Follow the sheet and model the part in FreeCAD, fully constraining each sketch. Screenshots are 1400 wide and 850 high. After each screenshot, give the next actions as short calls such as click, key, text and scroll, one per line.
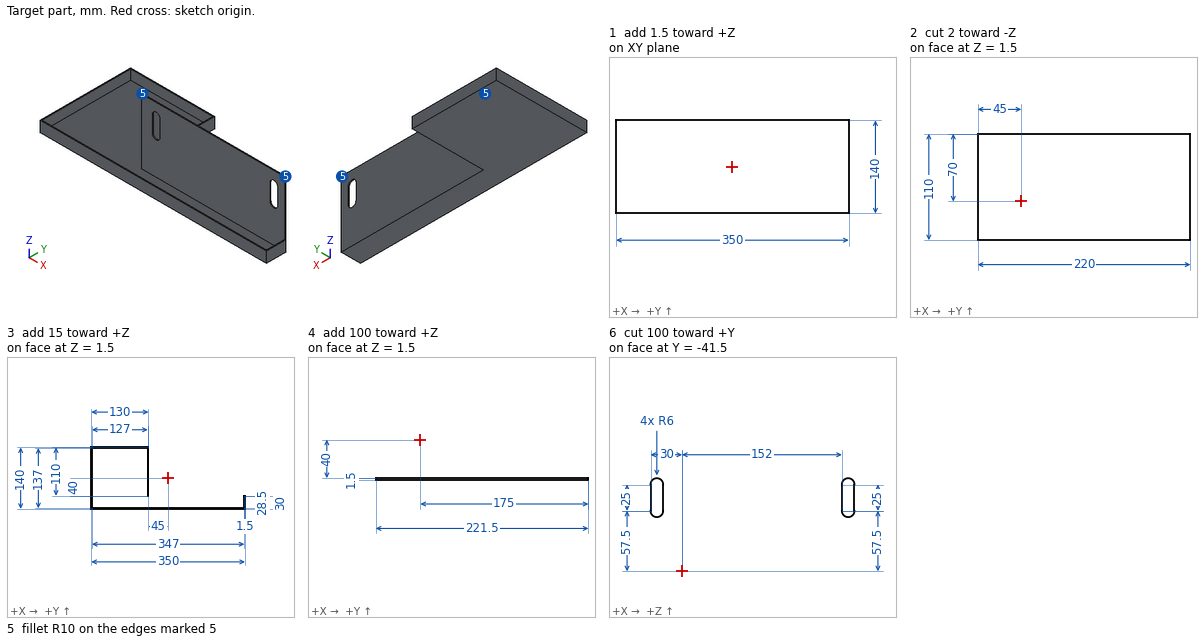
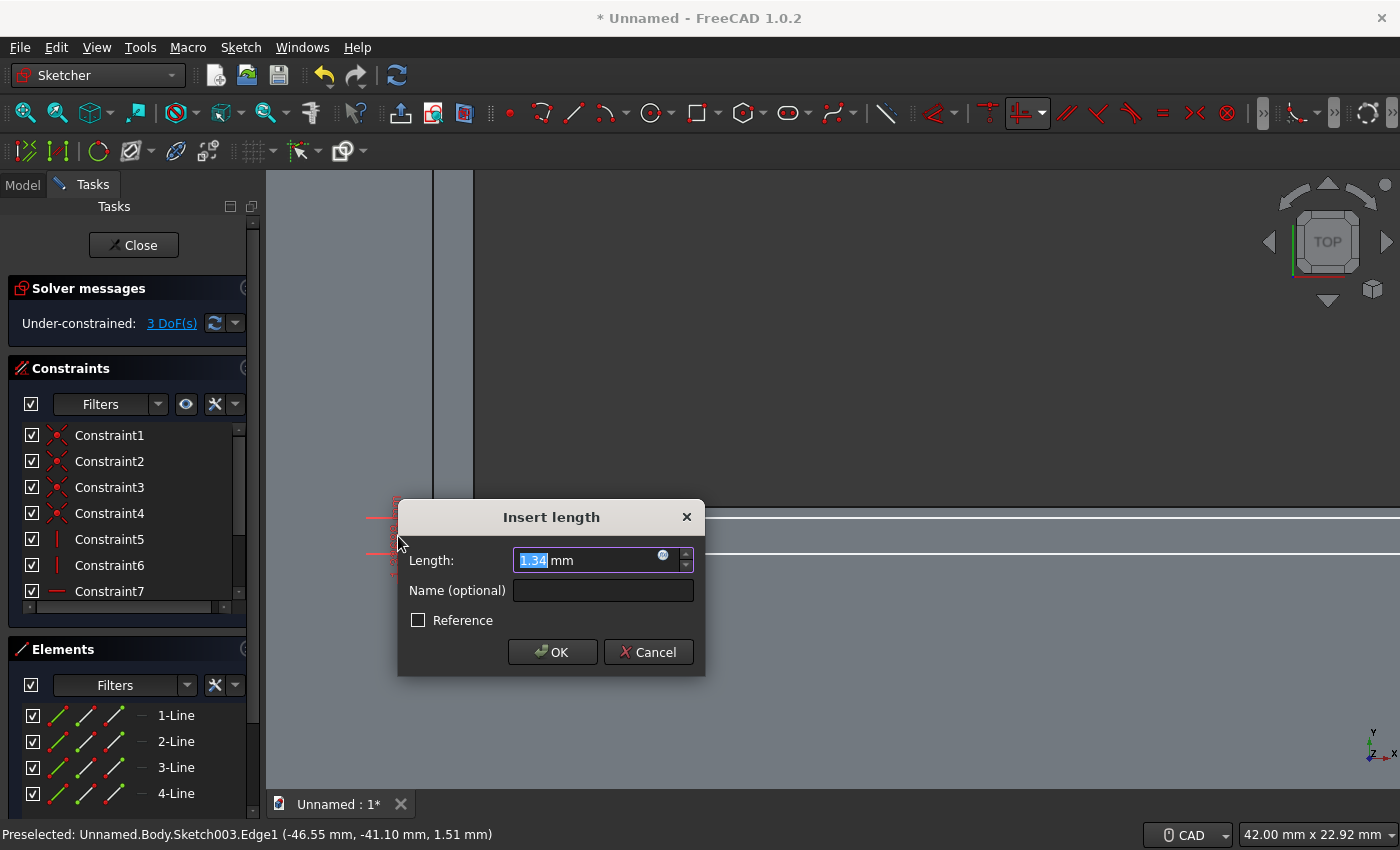
text(1.5)
key(Return)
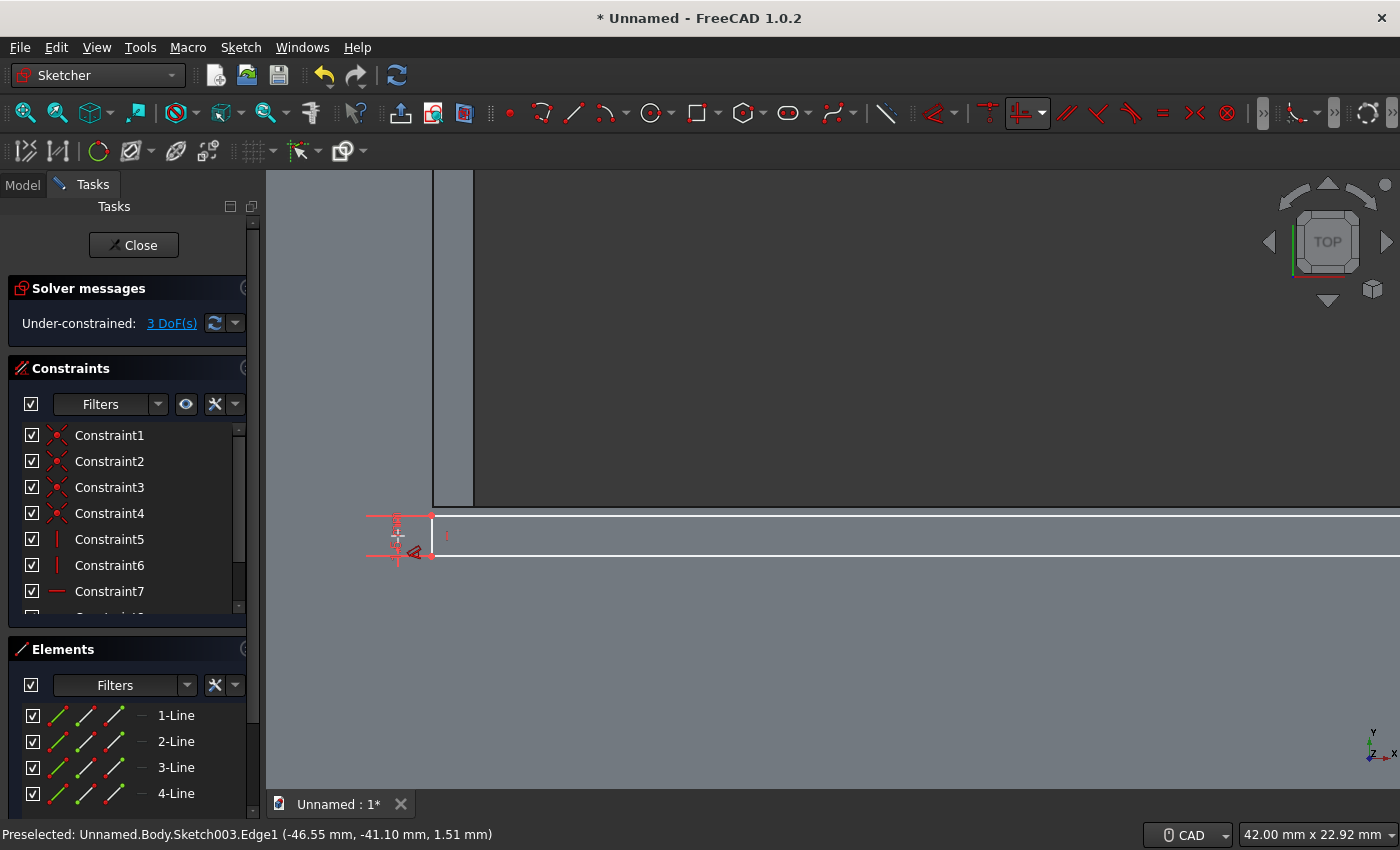
scroll(433, 541, down, 11)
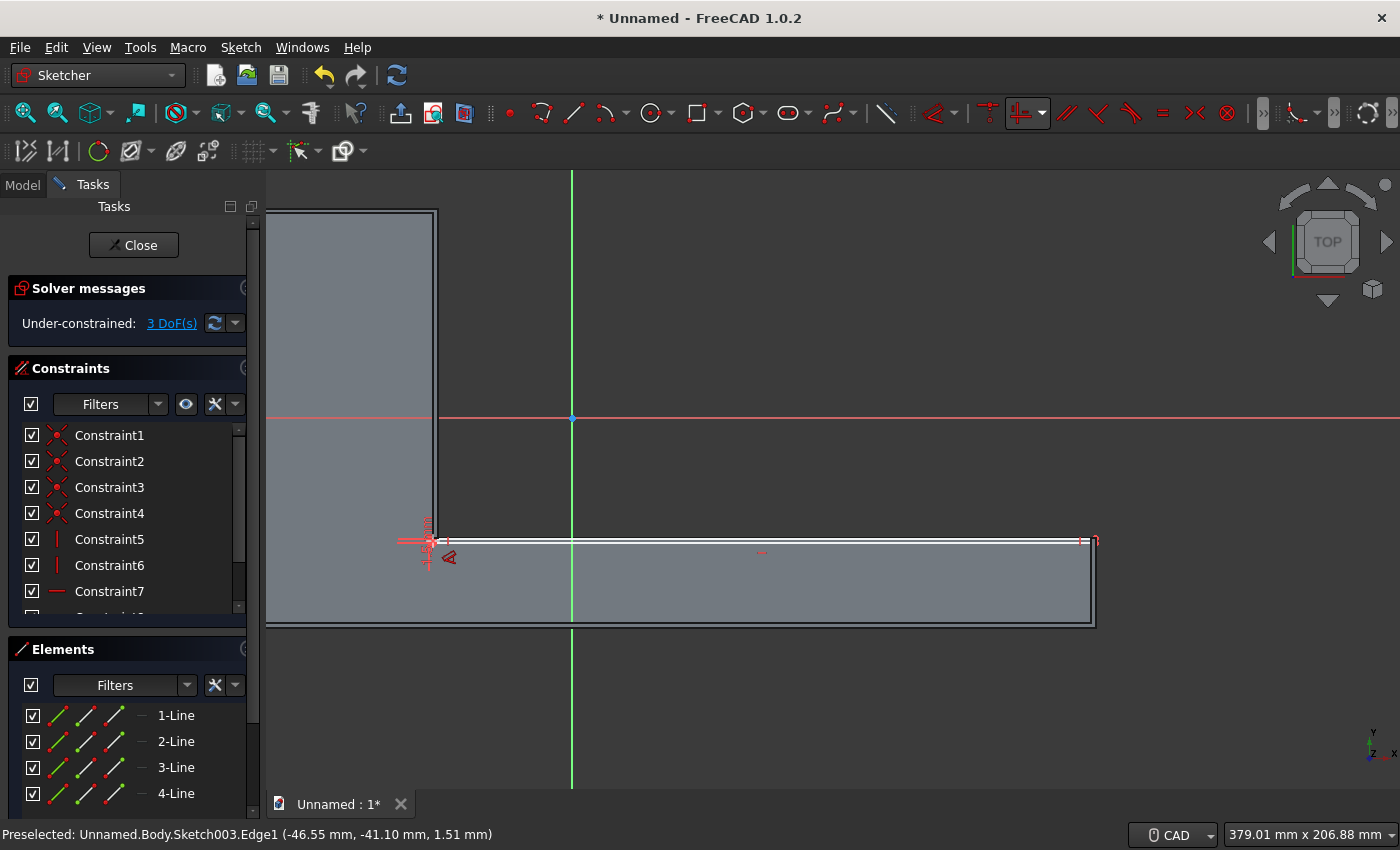
scroll(433, 539, up, 6)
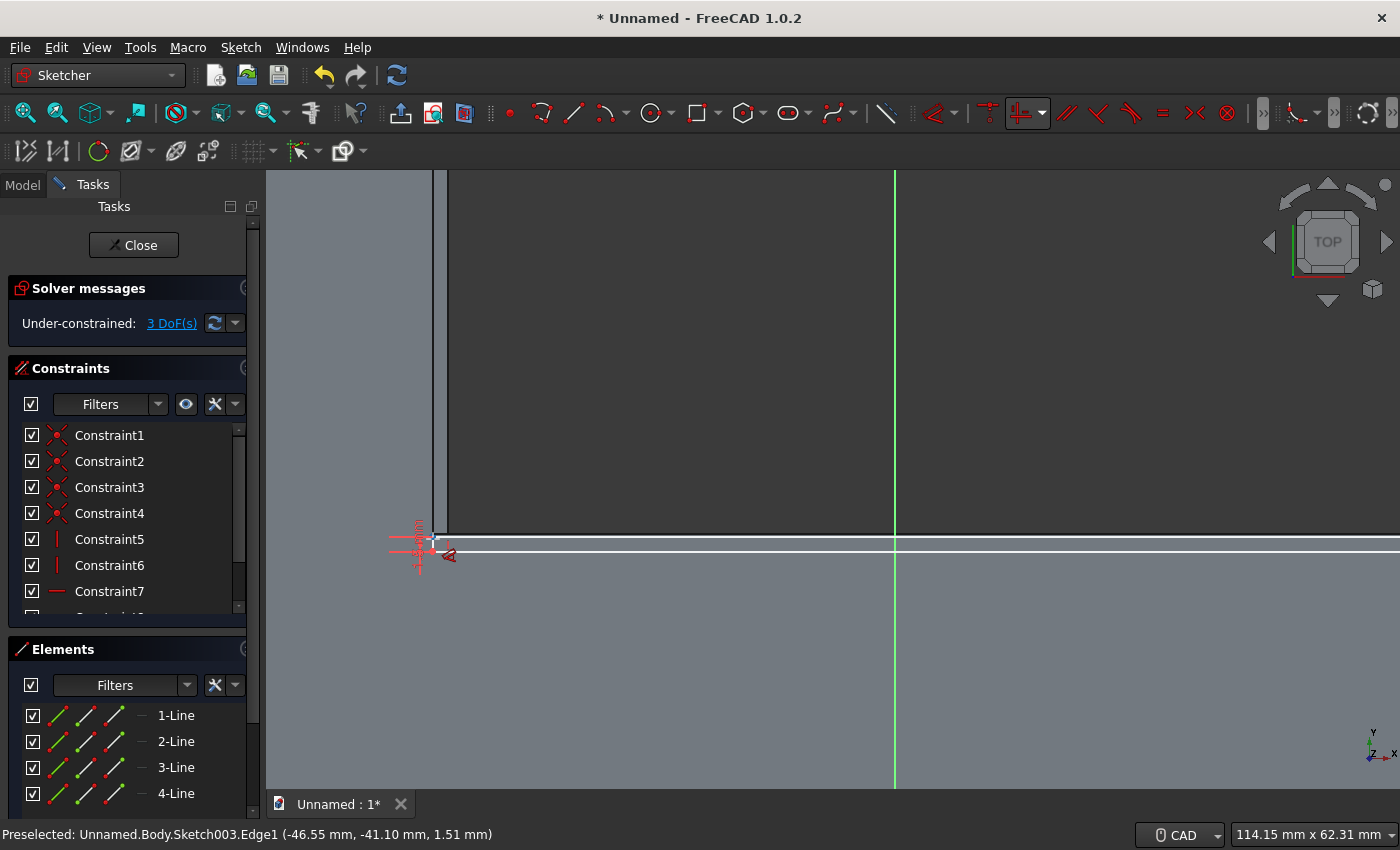
click(433, 537)
click(399, 367)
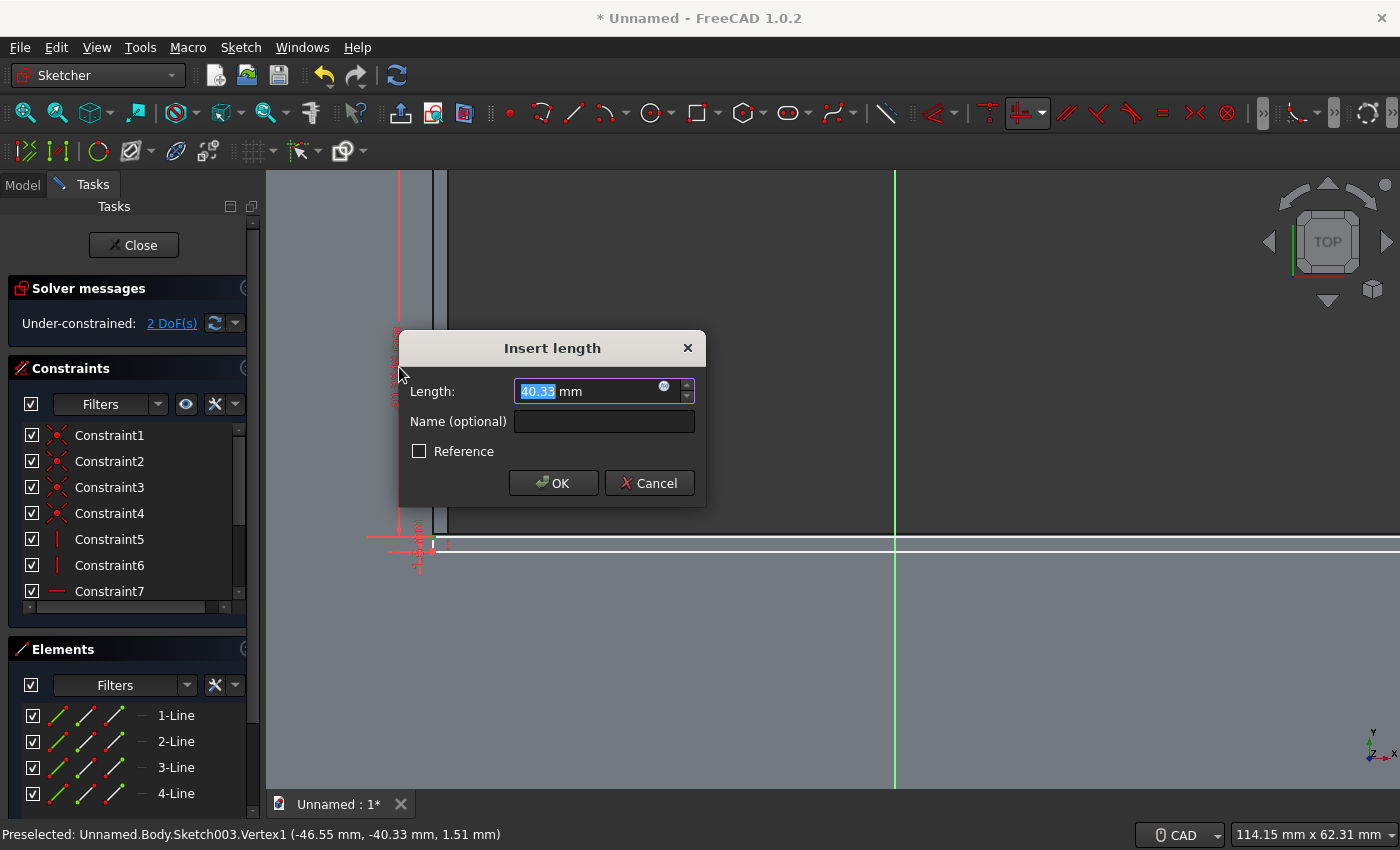
text(40)
key(Return)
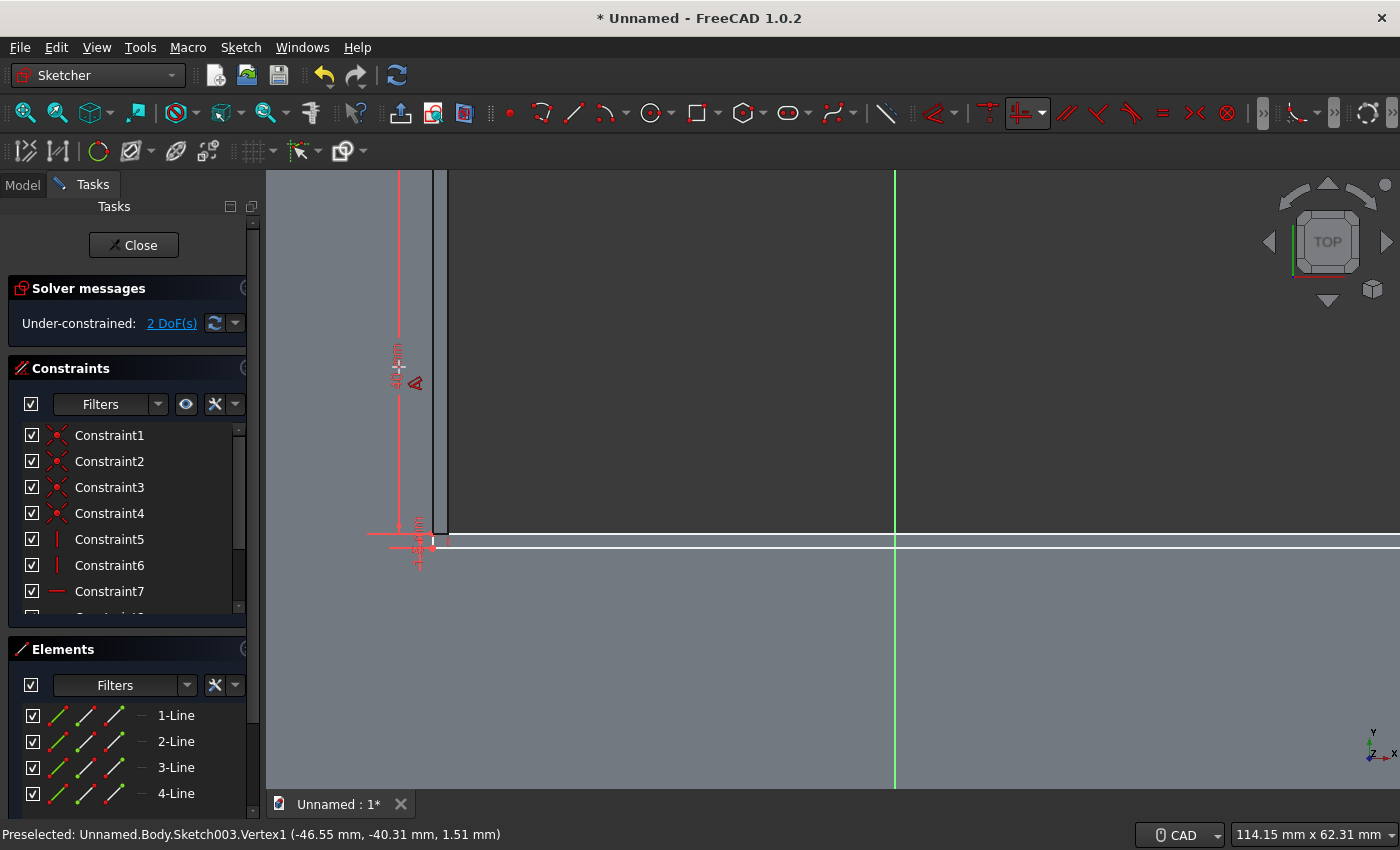
scroll(433, 539, down, 6)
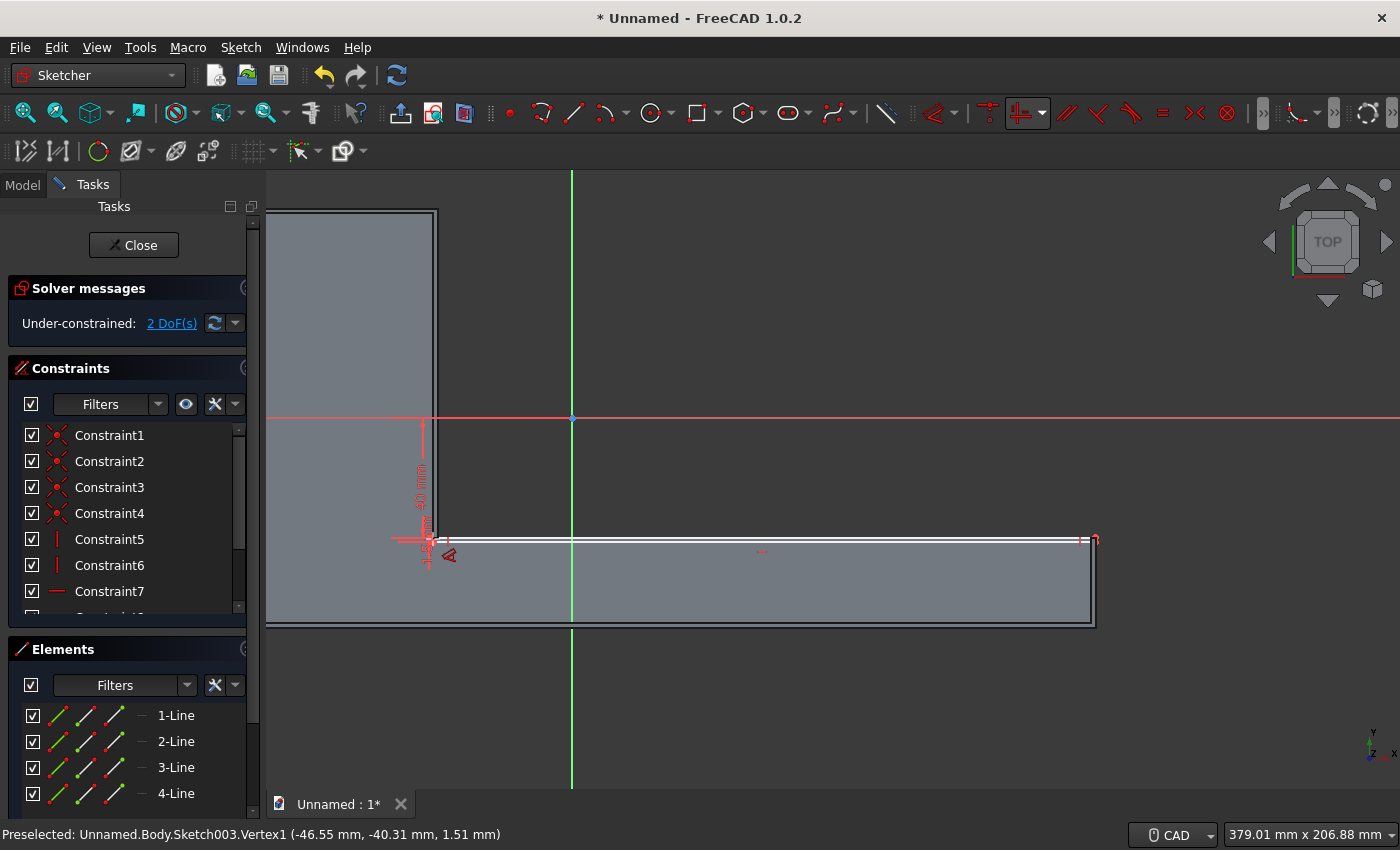
scroll(1096, 542, up, 6)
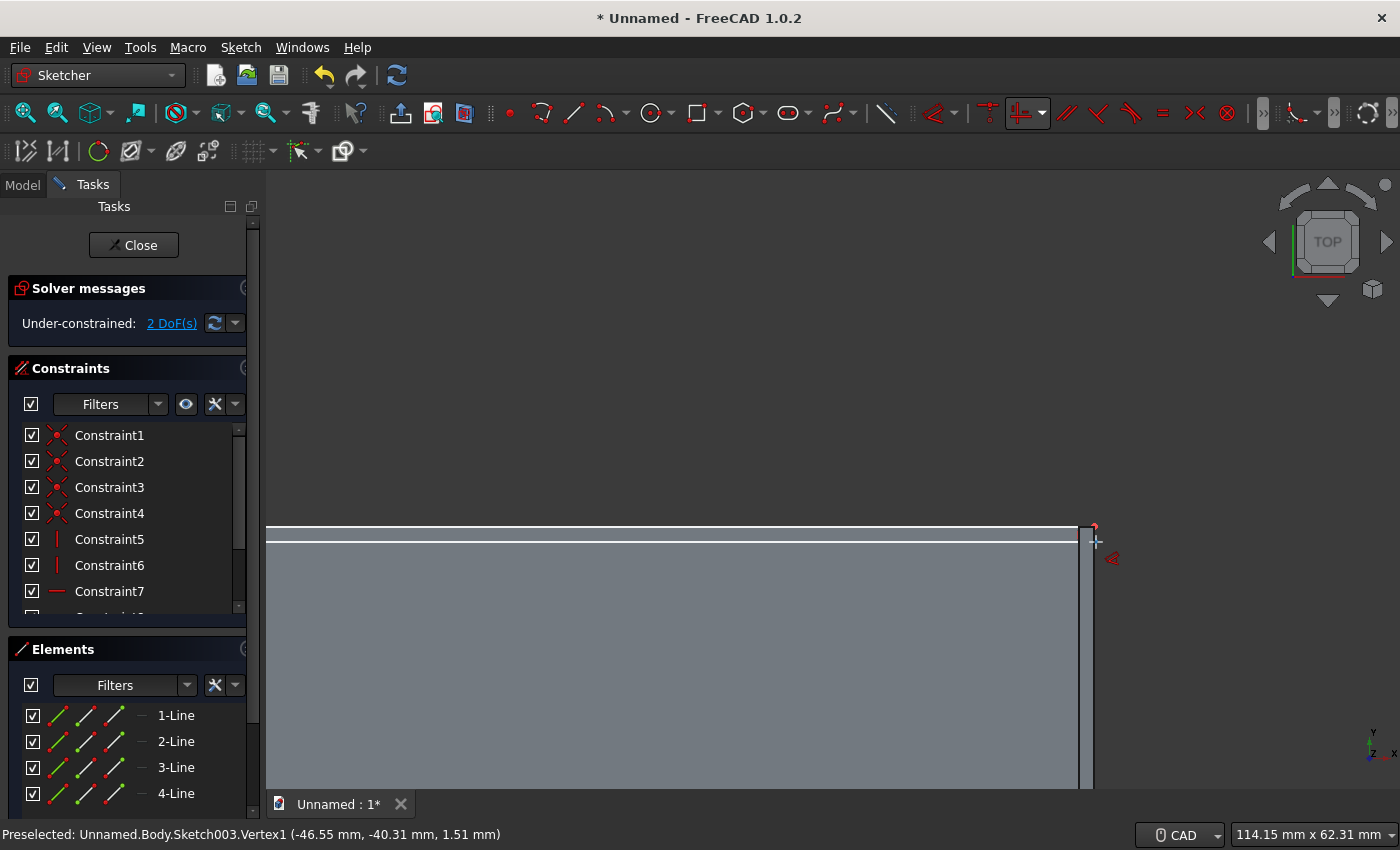
click(1094, 542)
click(694, 576)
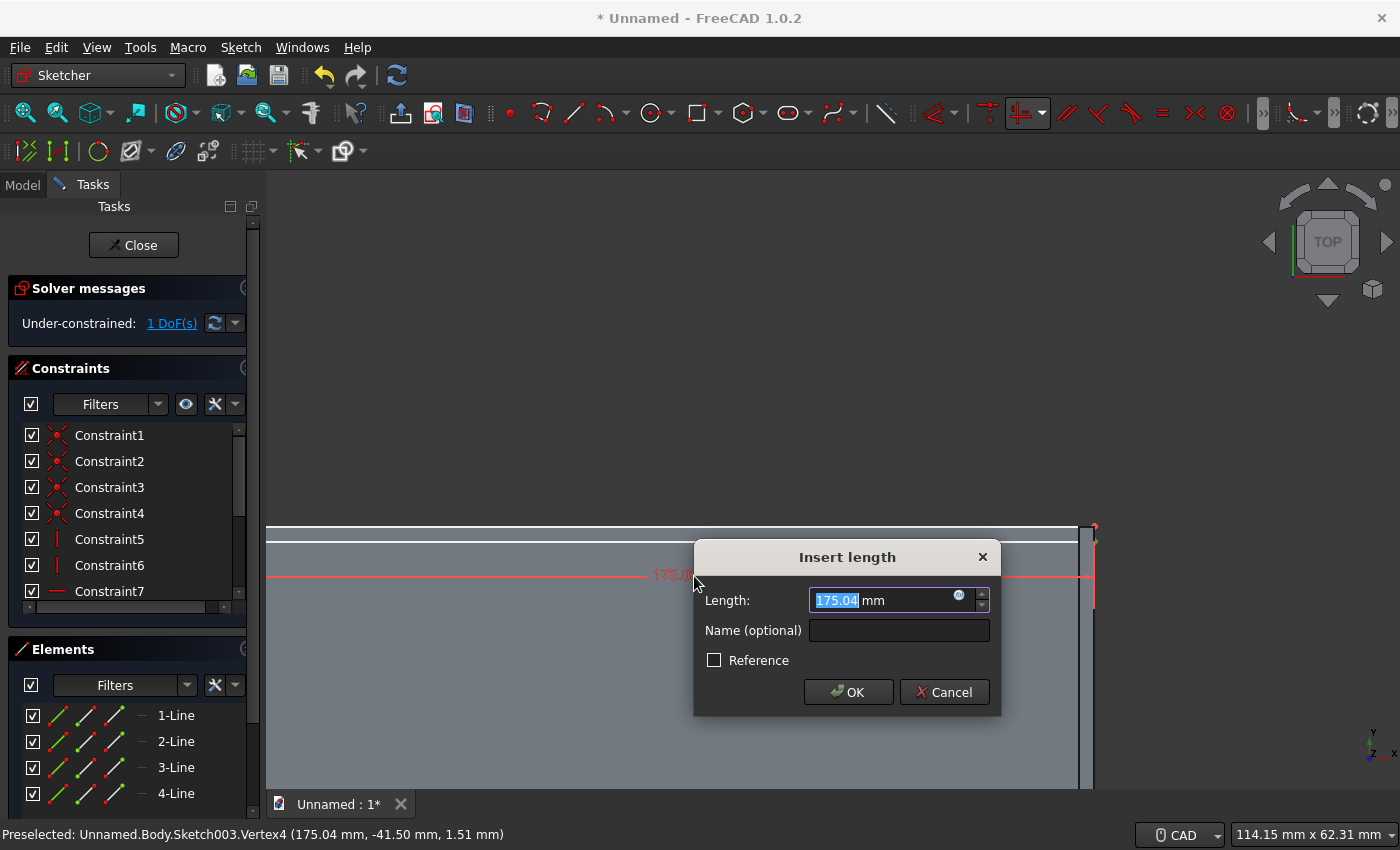
text(175)
key(Return)